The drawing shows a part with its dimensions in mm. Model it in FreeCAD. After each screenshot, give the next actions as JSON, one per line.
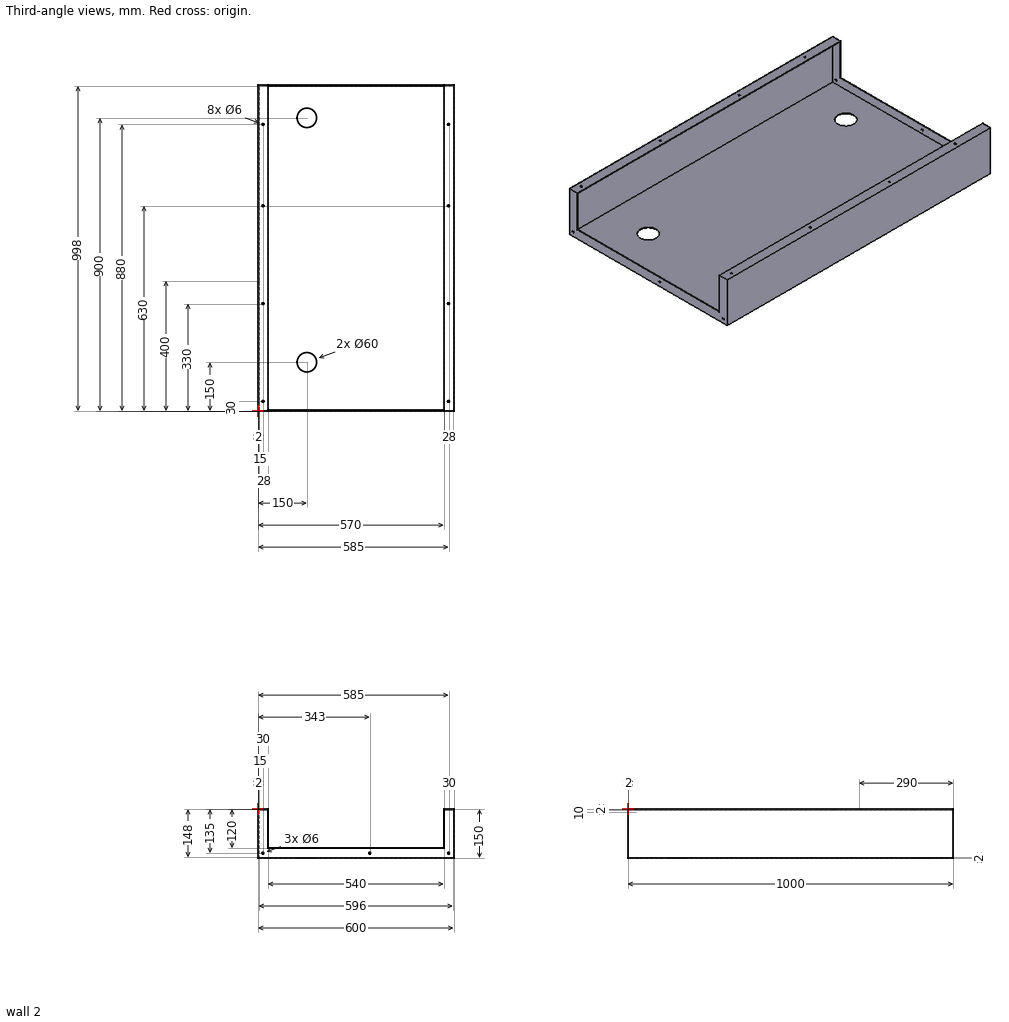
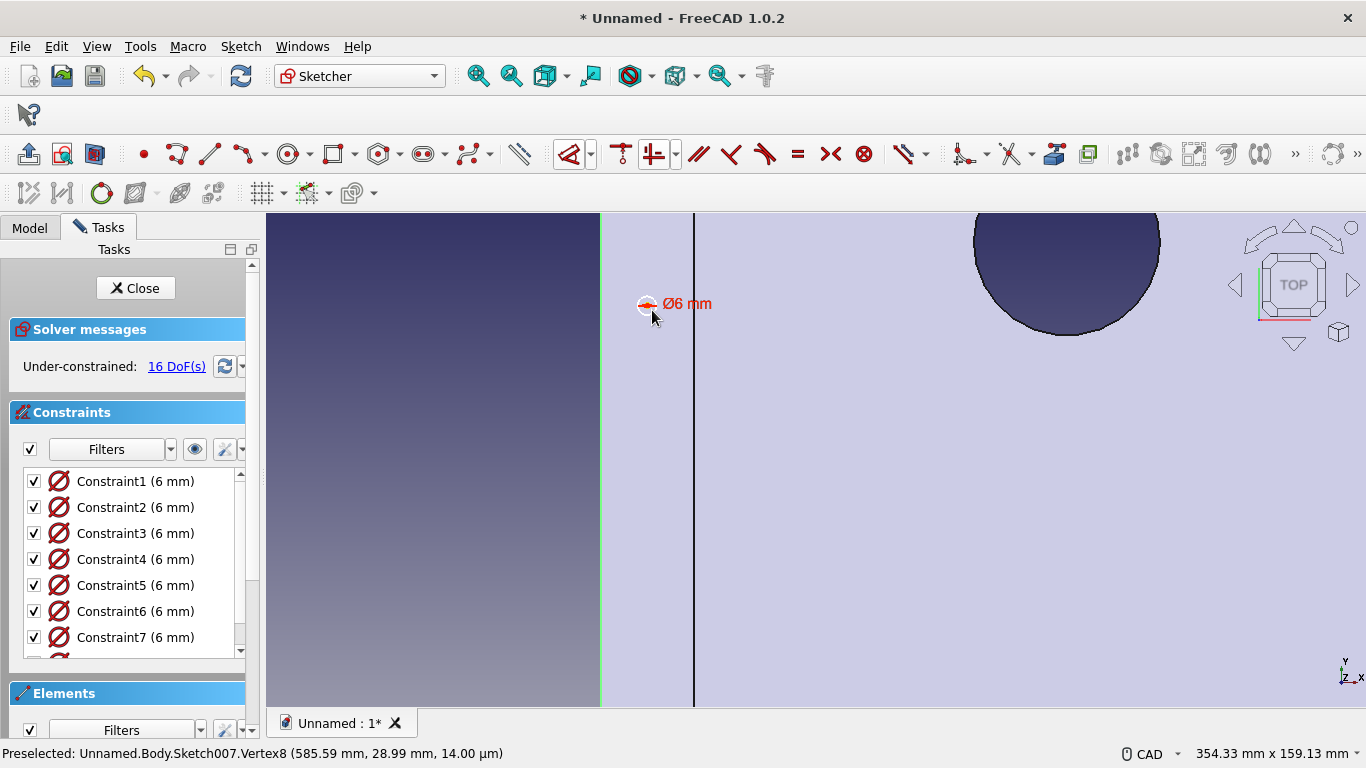
{"action": "left_click", "coordinate": [647, 306]}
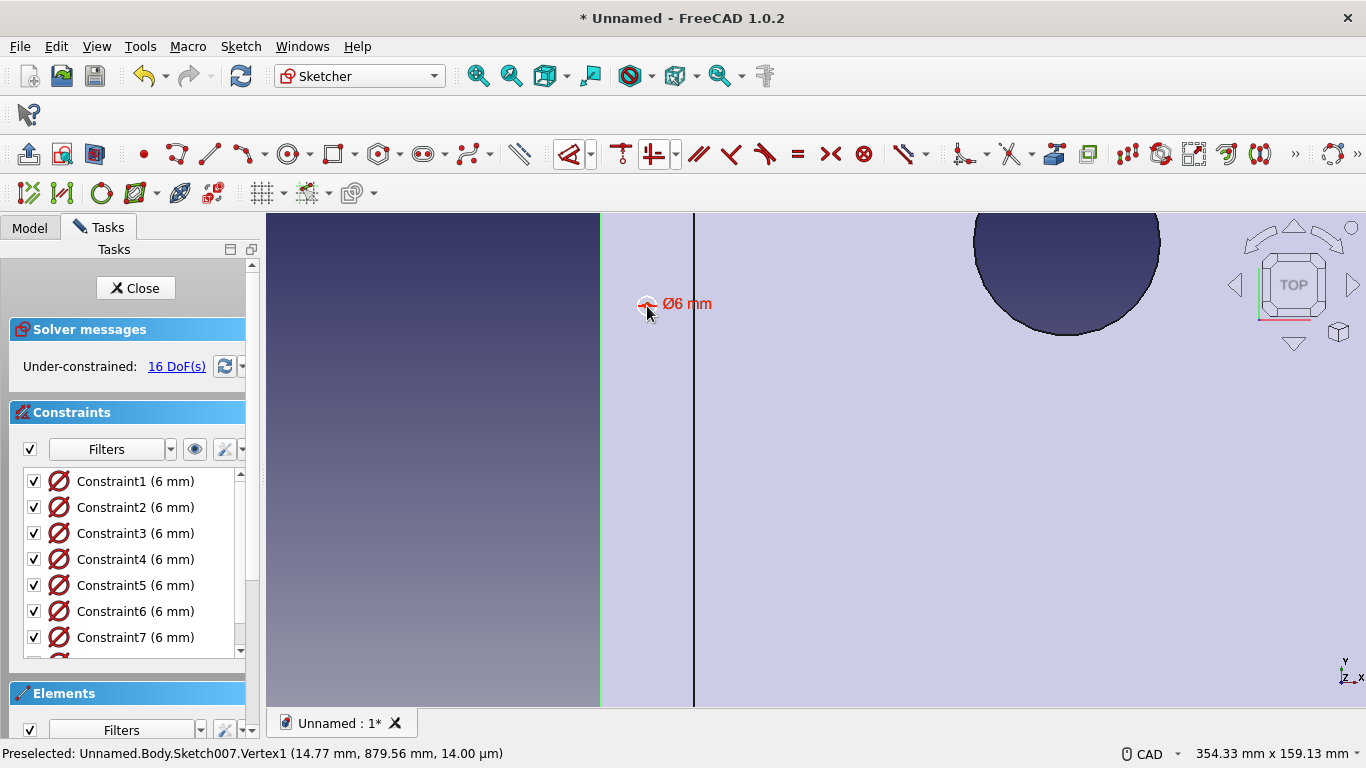
{"action": "key", "text": "l"}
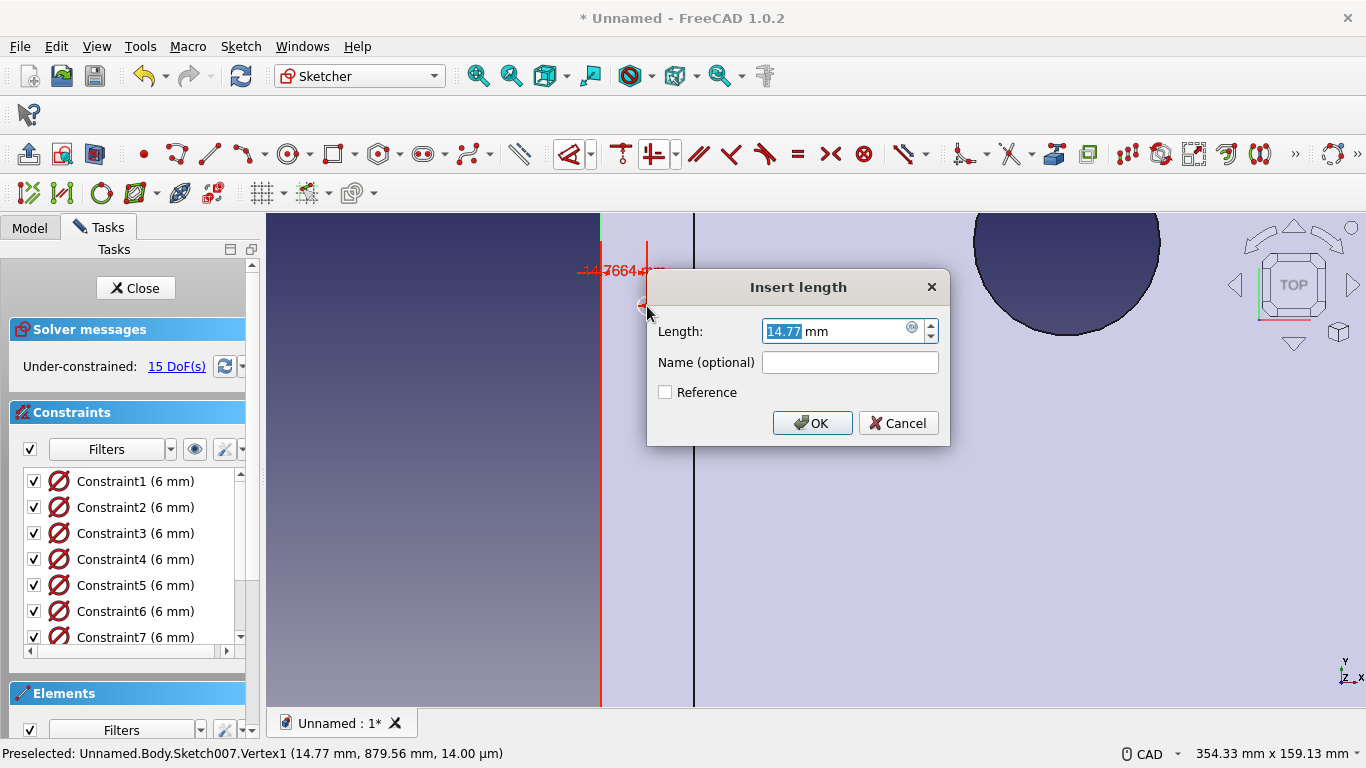
{"action": "type", "text": "15"}
{"action": "key", "text": "Return"}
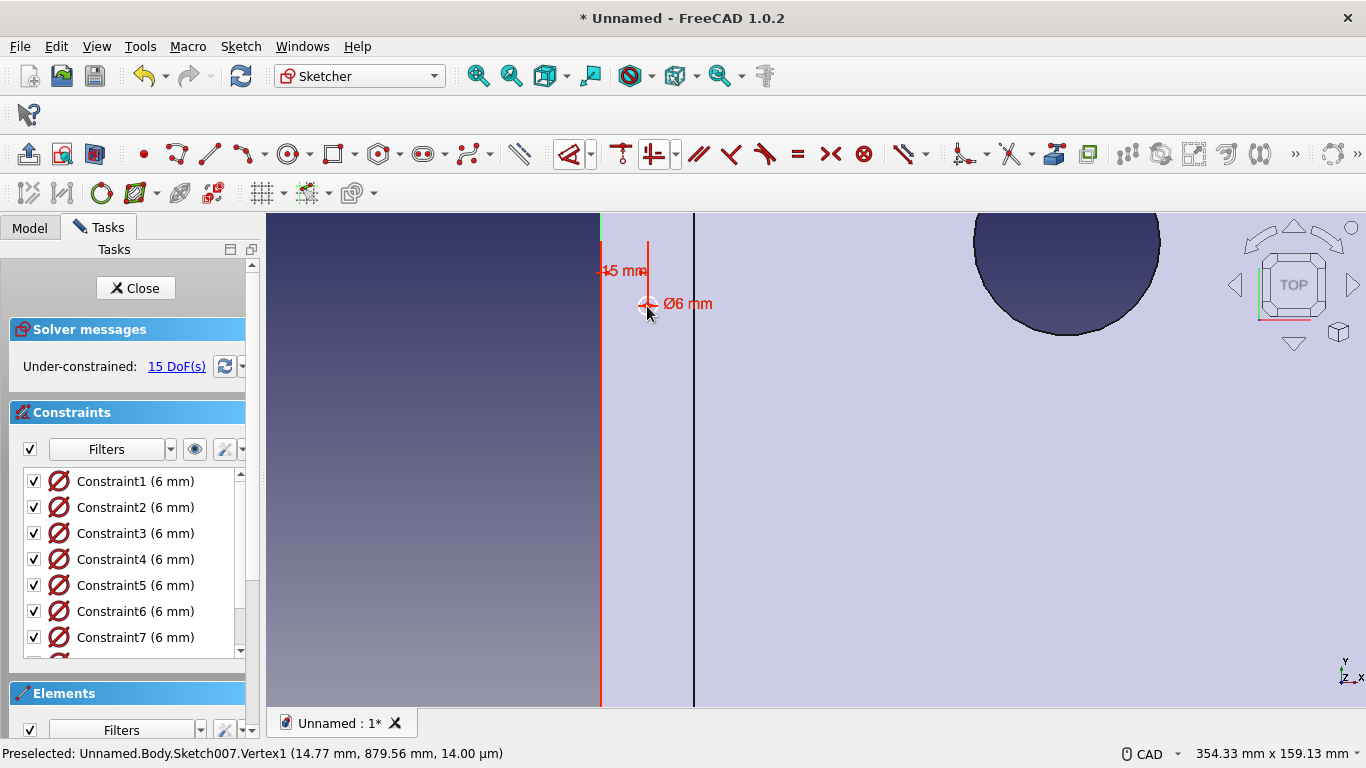
{"action": "scroll", "coordinate": [652, 310], "scroll_direction": "down", "scroll_amount": 11}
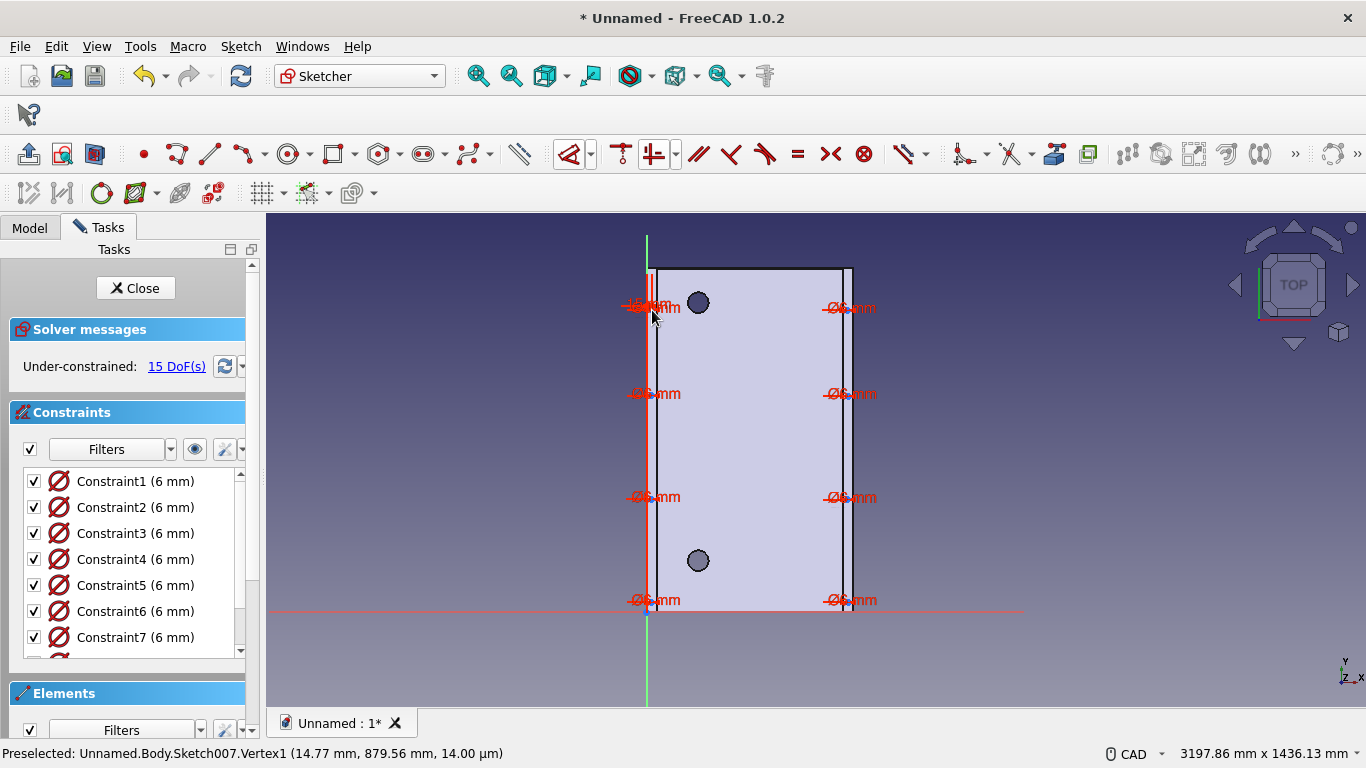
{"action": "scroll", "coordinate": [652, 602], "scroll_direction": "up", "scroll_amount": 11}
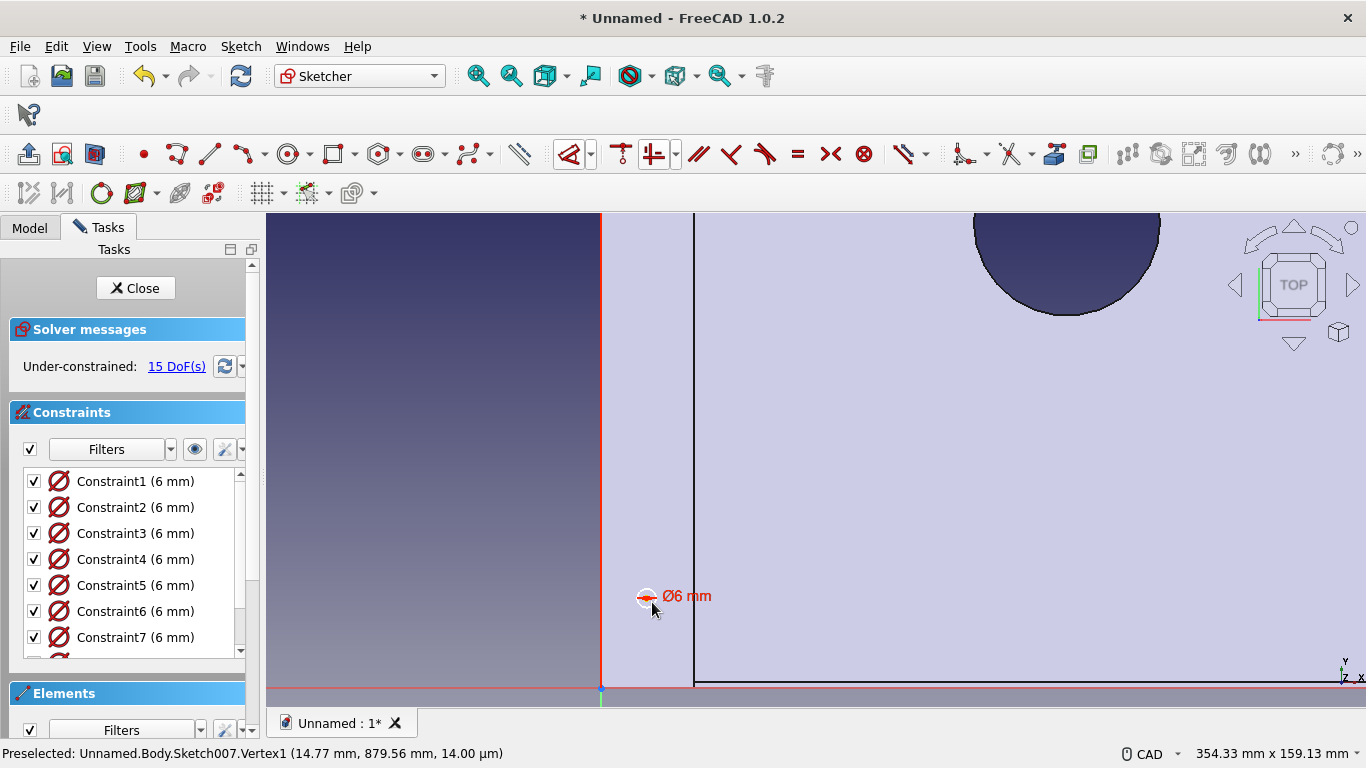
{"action": "left_click", "coordinate": [647, 598]}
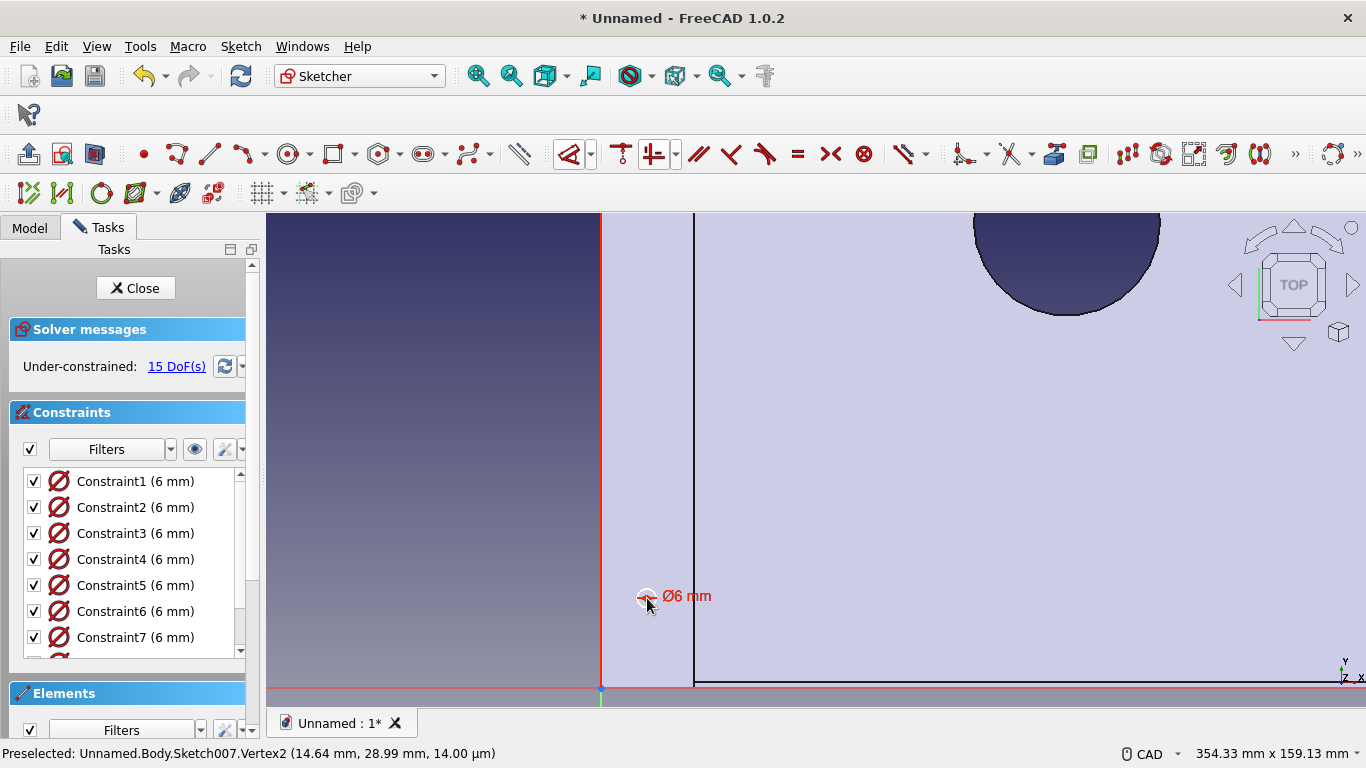
{"action": "left_click", "coordinate": [590, 154]}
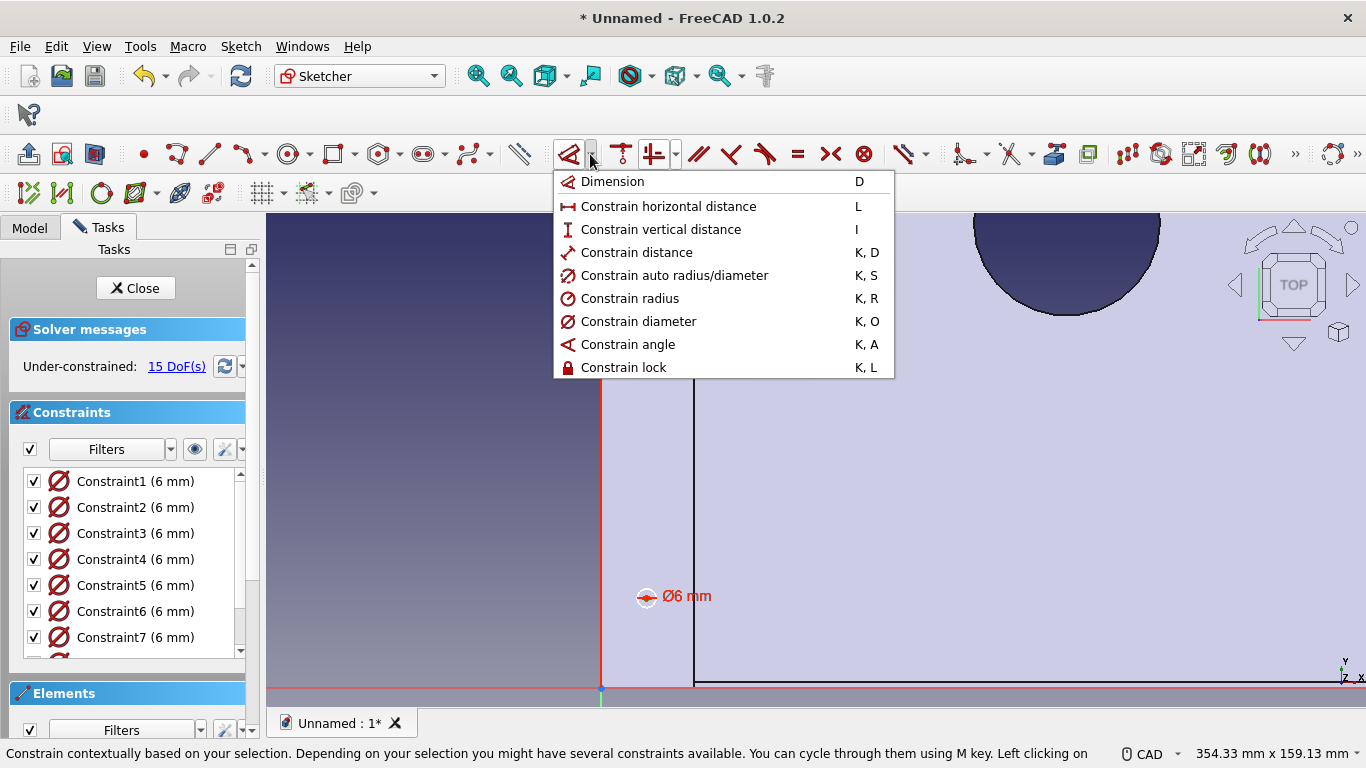
{"action": "left_click", "coordinate": [724, 206]}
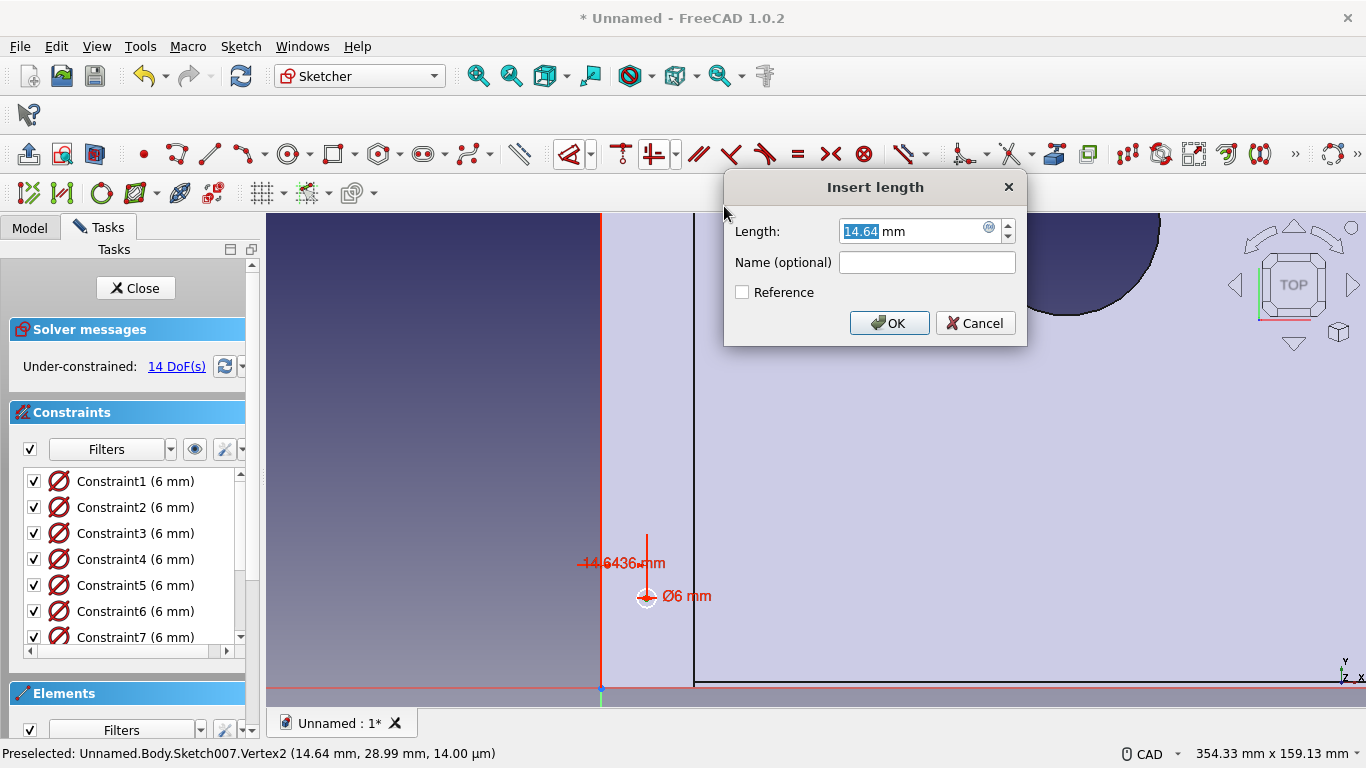
{"action": "type", "text": "15"}
{"action": "key", "text": "Return"}